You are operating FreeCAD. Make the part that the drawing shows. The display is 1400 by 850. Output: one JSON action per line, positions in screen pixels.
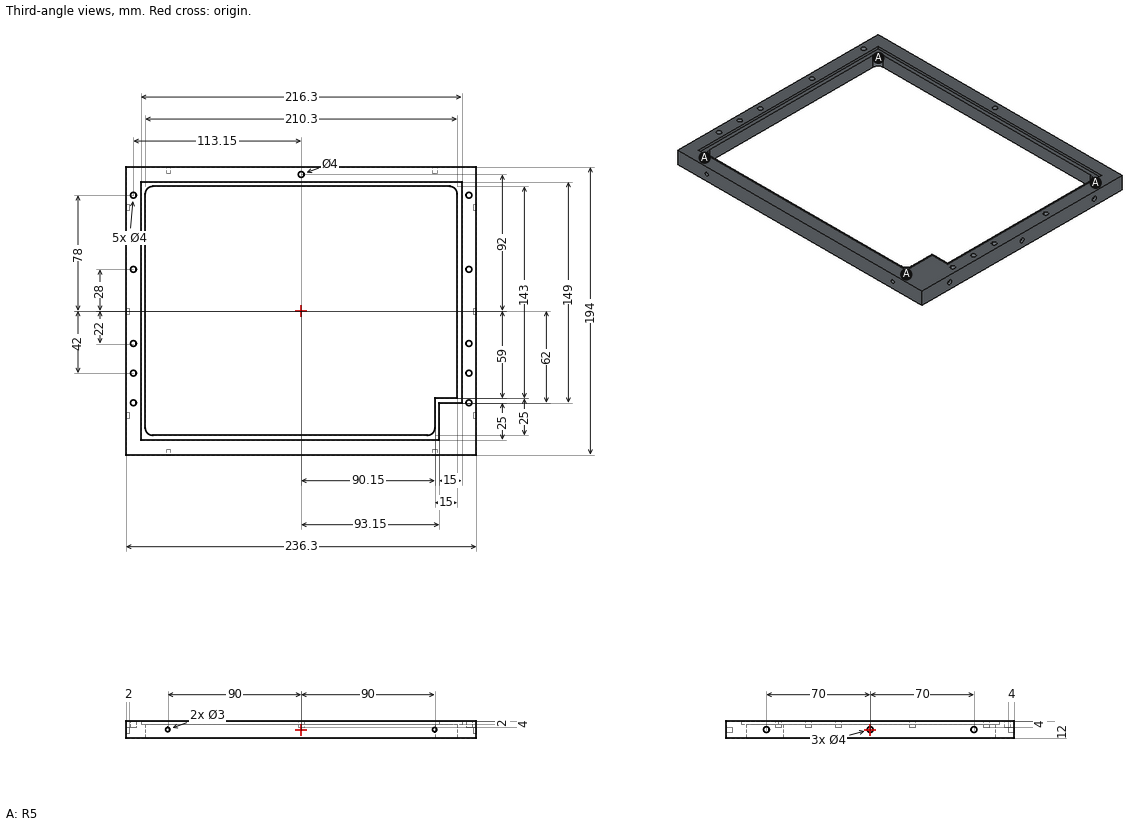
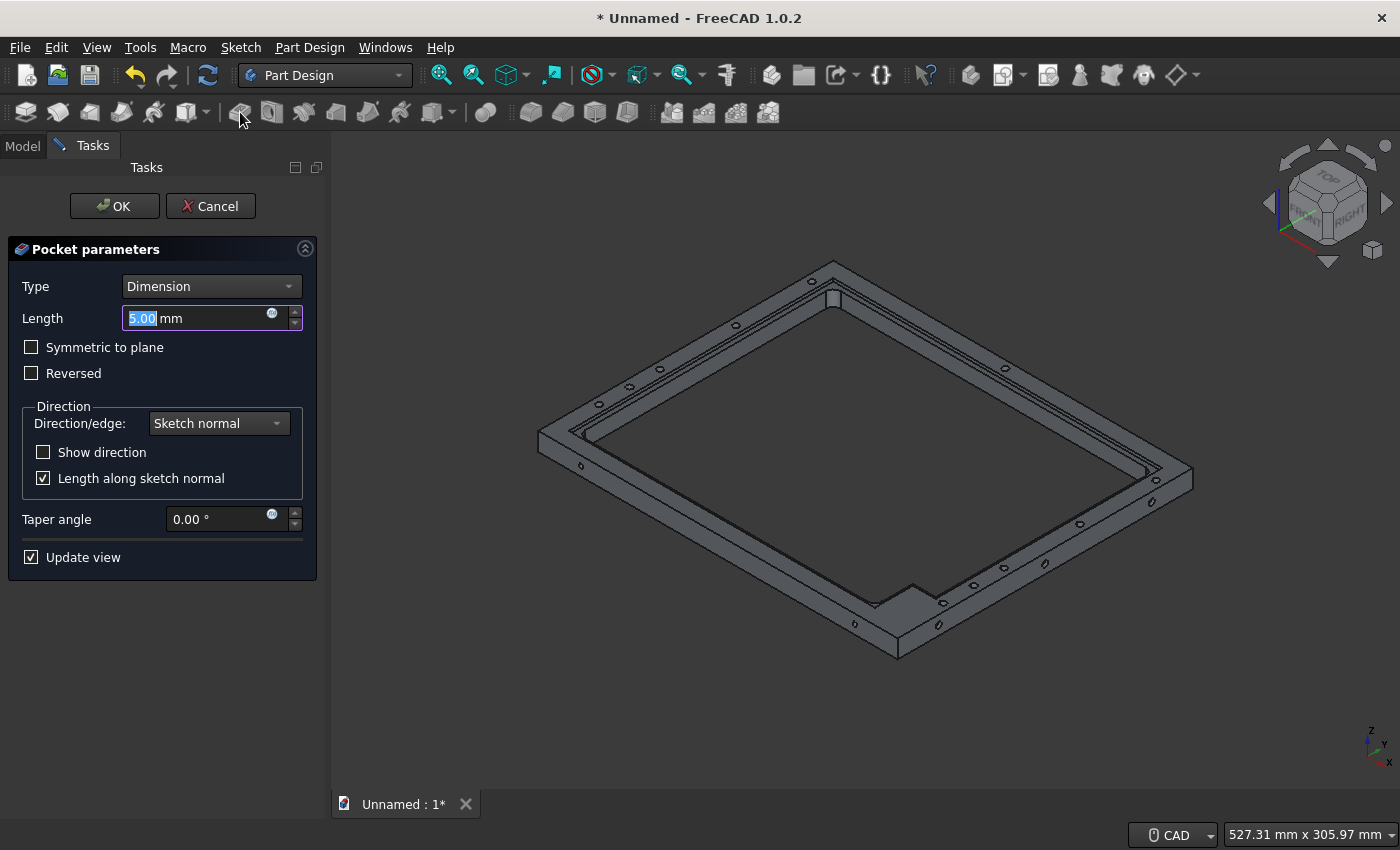
{"action": "type", "text": "4"}
{"action": "key", "text": "Tab"}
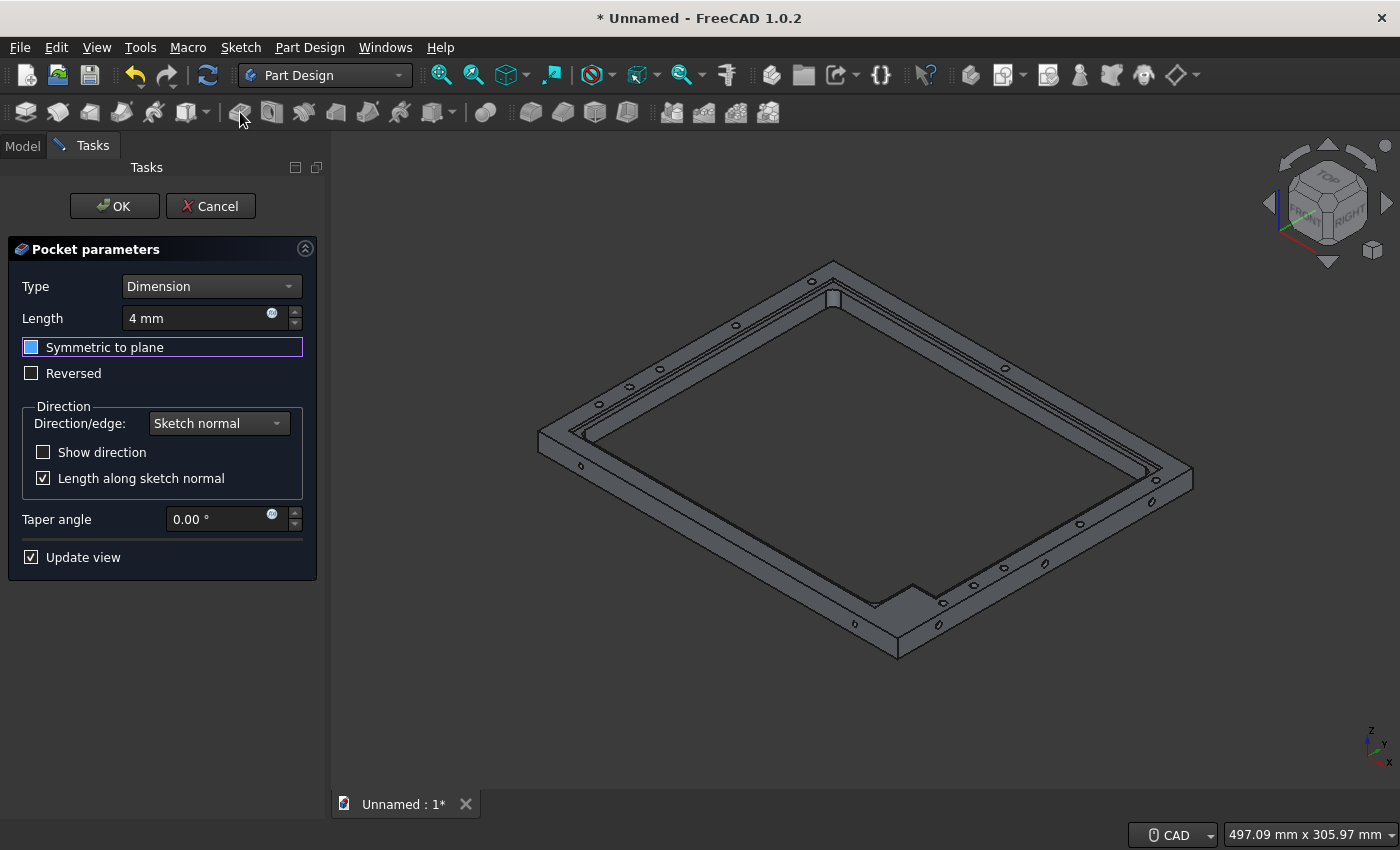
{"action": "left_click", "coordinate": [115, 206]}